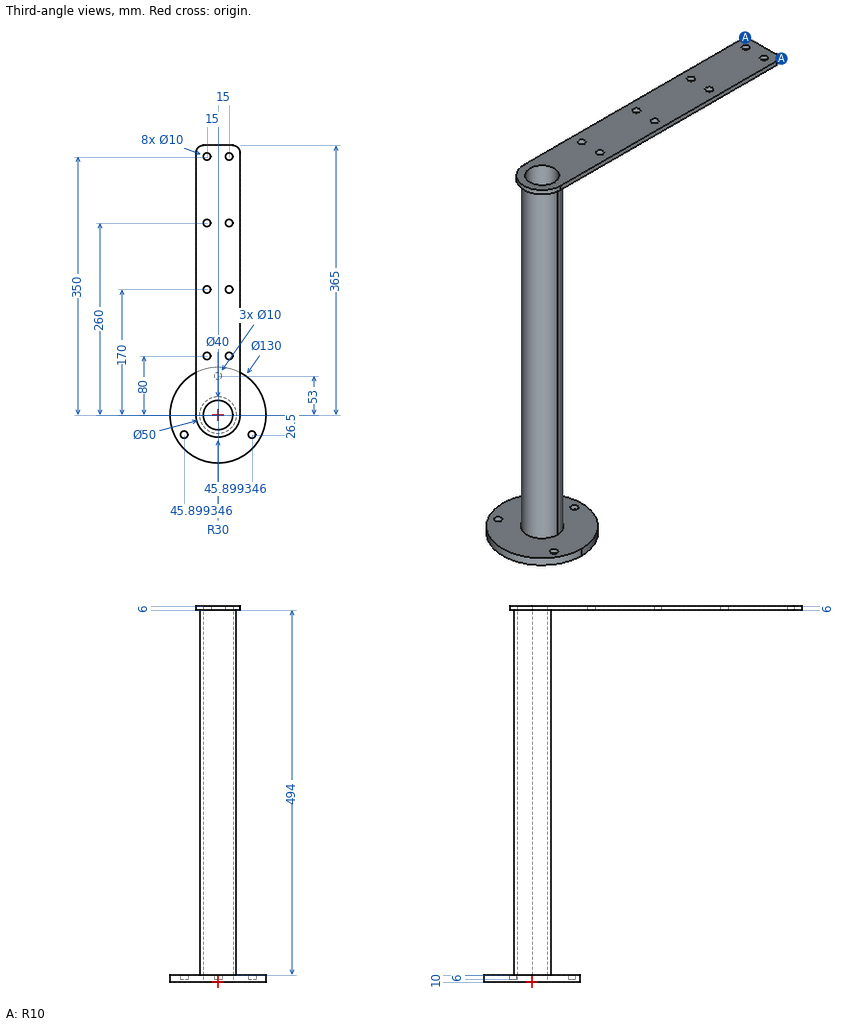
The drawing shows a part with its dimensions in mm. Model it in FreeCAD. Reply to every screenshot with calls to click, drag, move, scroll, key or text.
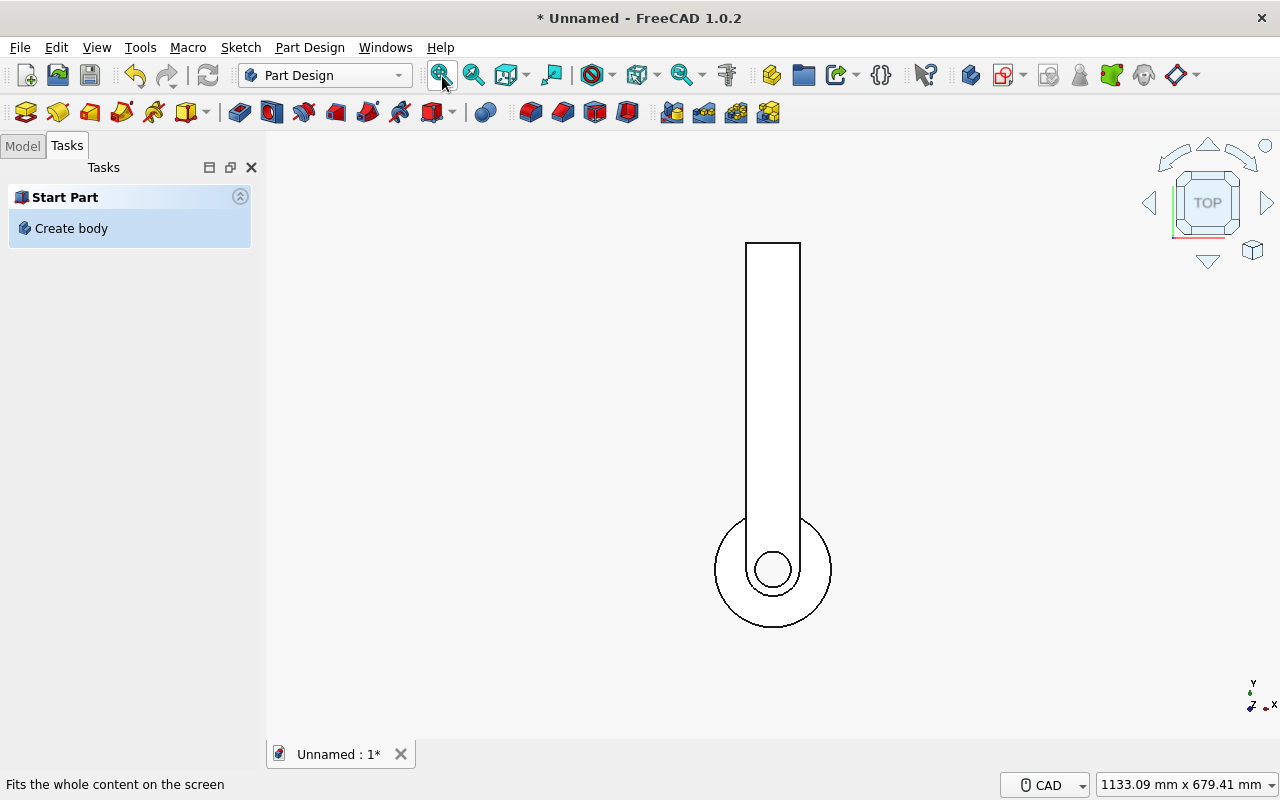
scroll(800, 242, up, 11)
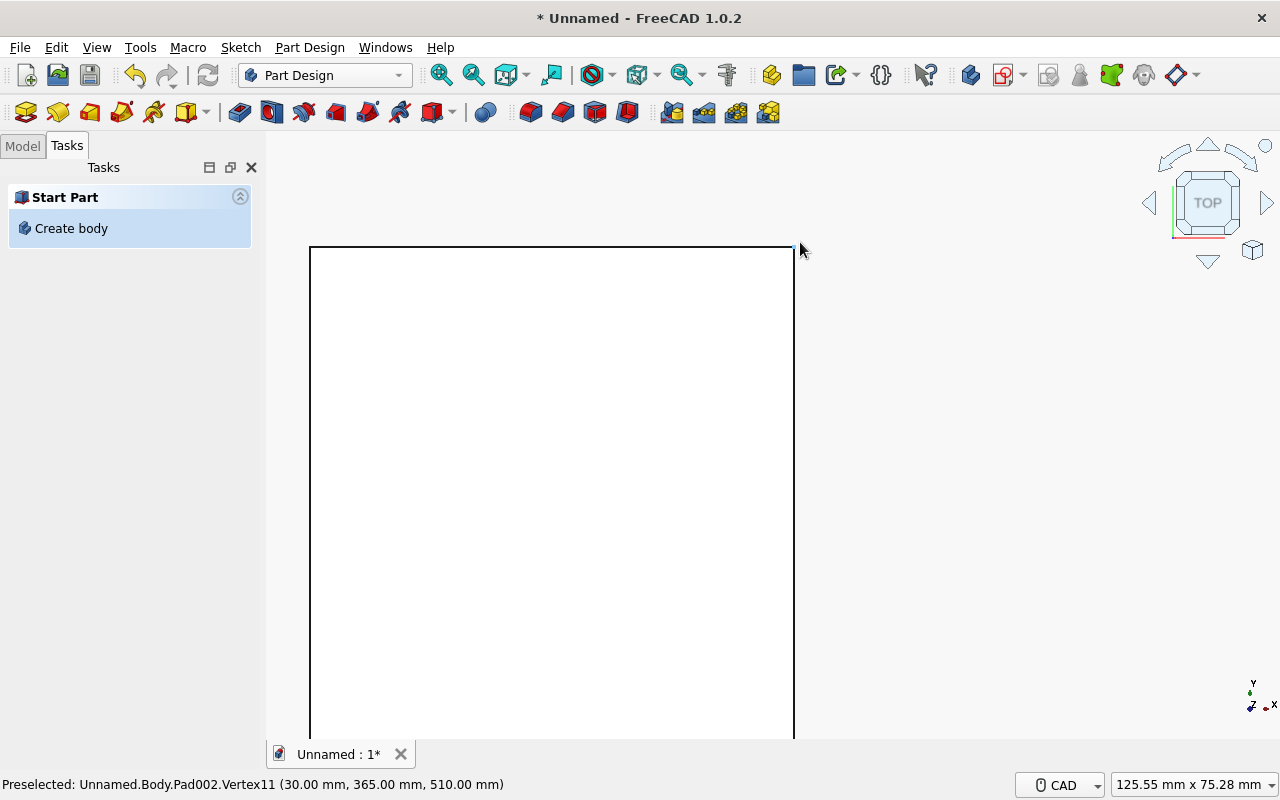
click(442, 76)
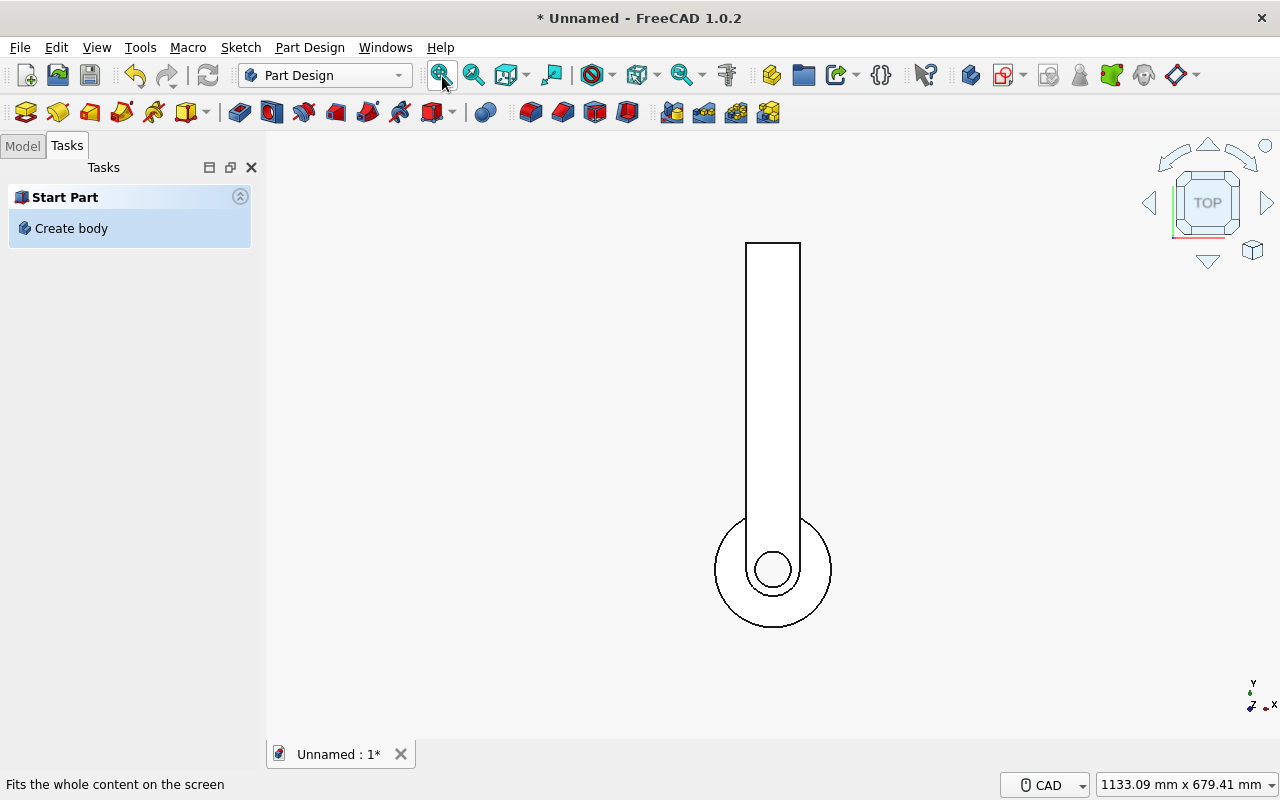
key(1)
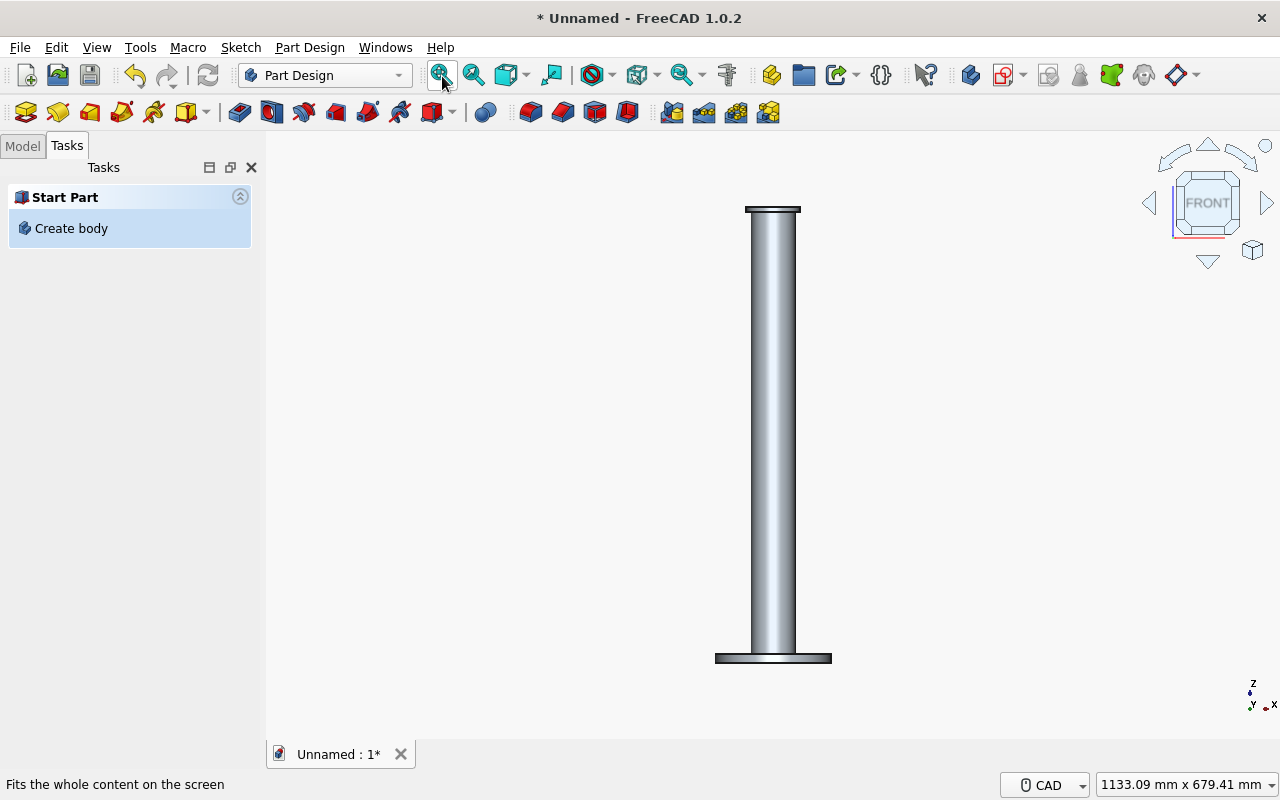
scroll(800, 208, up, 11)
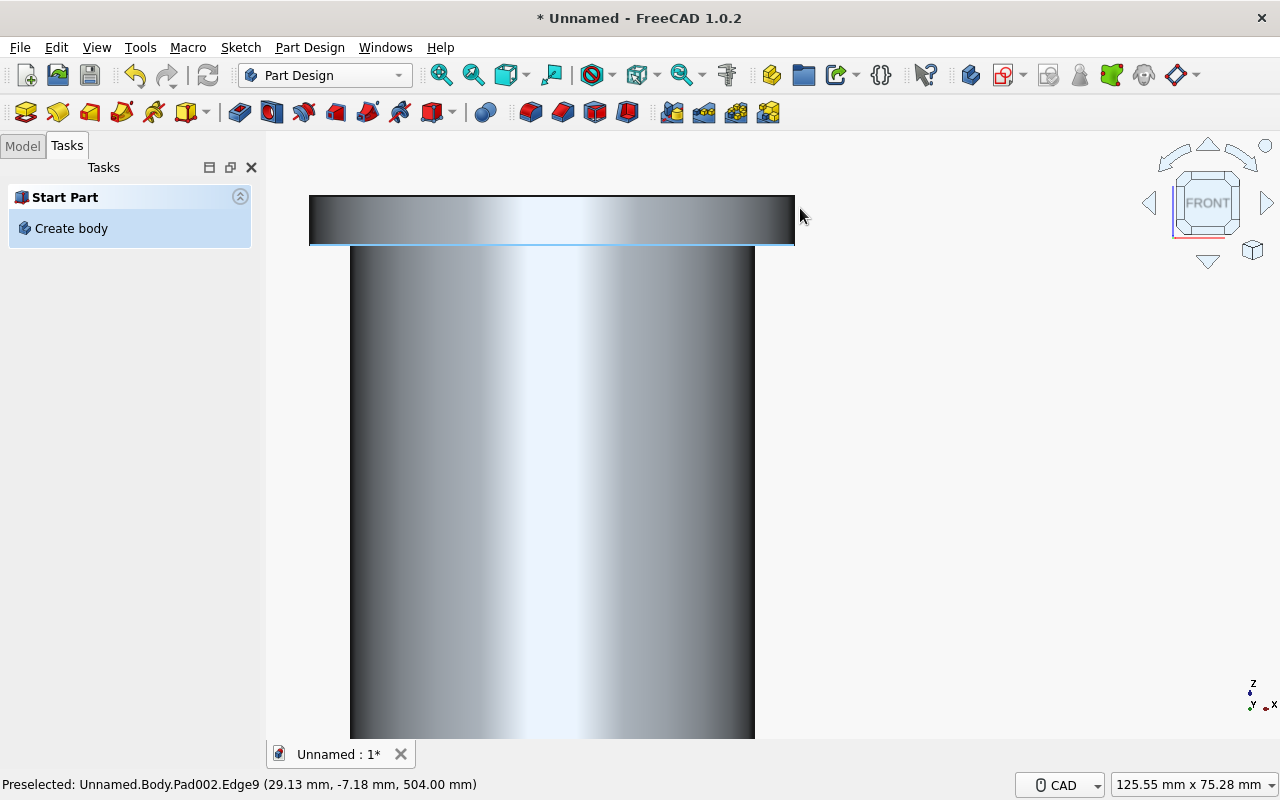
click(442, 76)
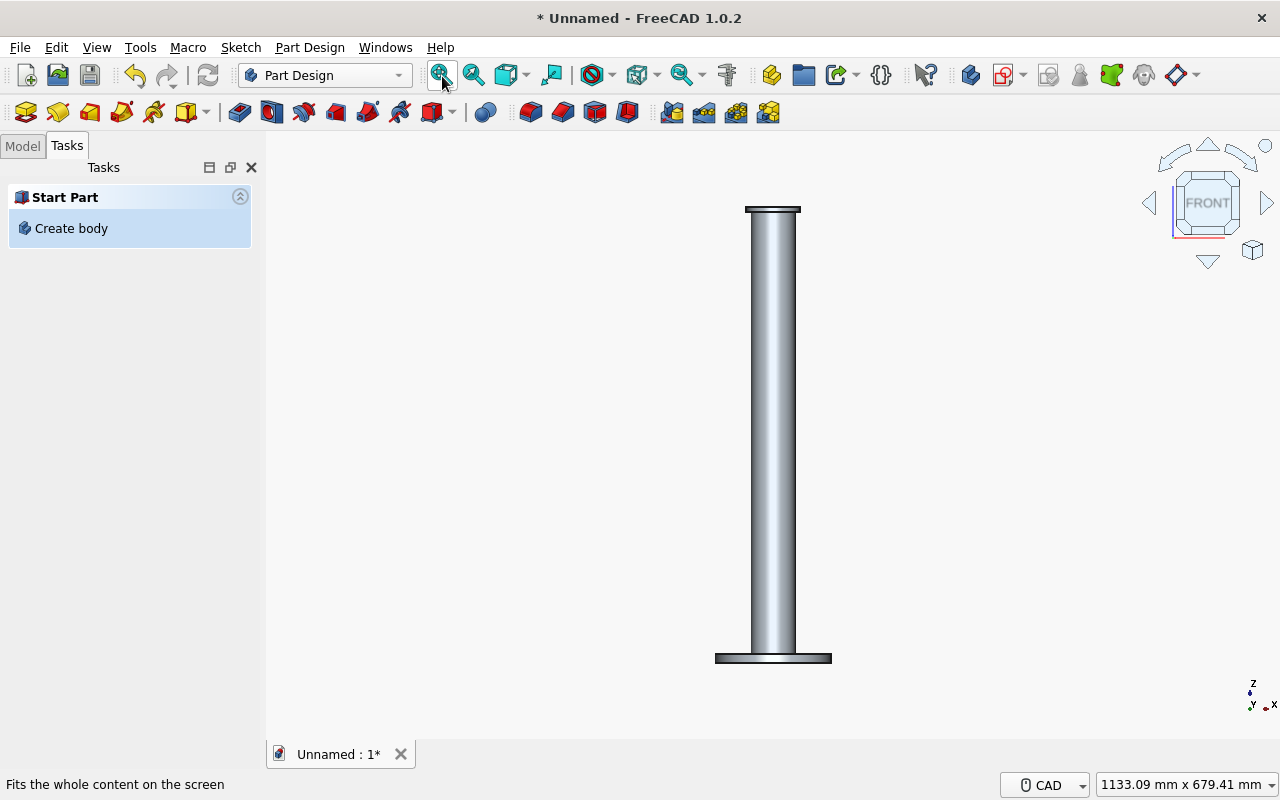
key(3)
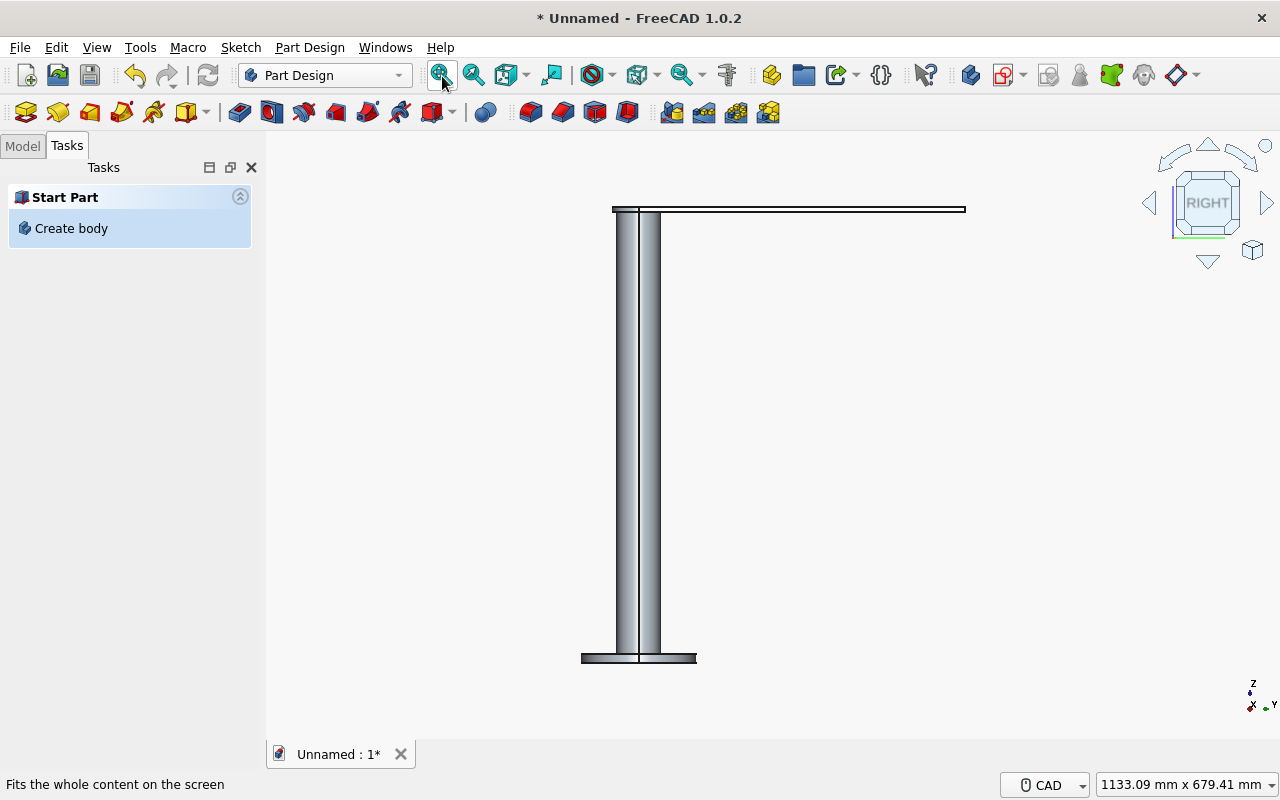
scroll(965, 208, up, 11)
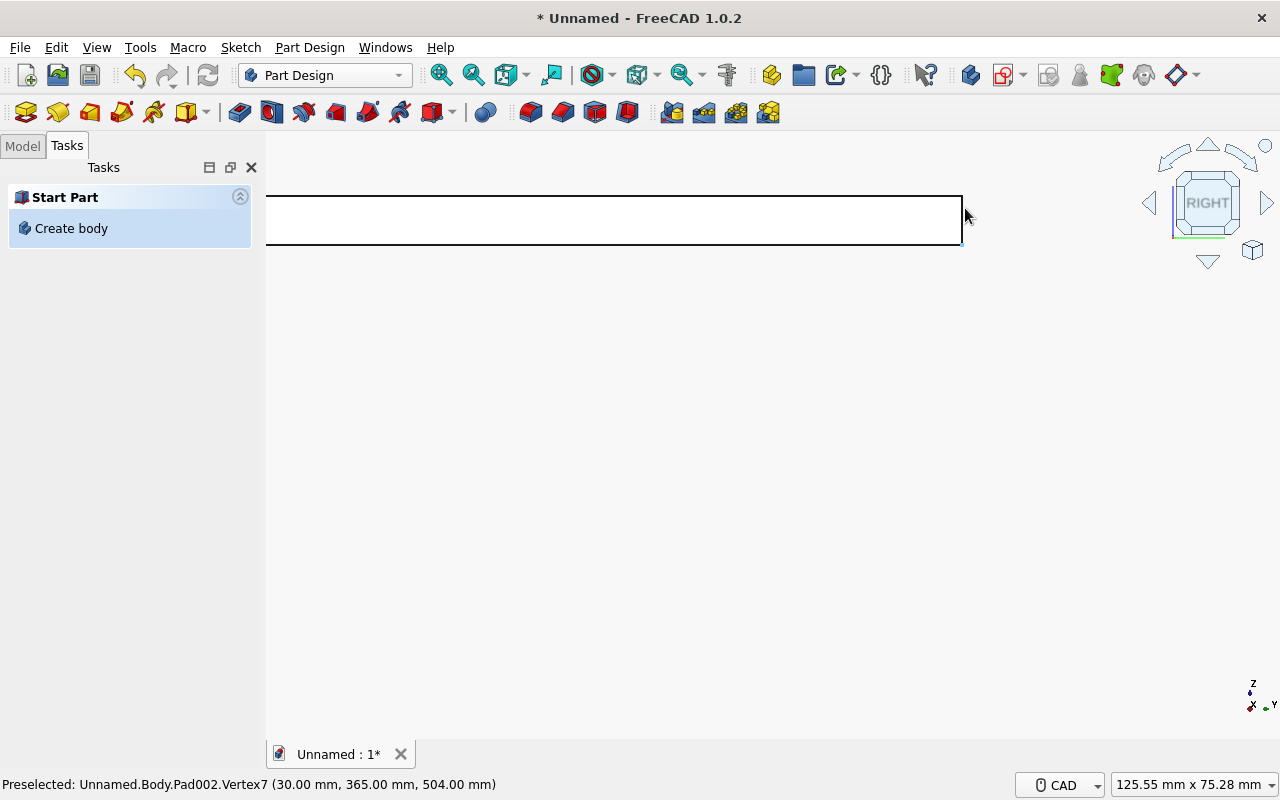
click(962, 219)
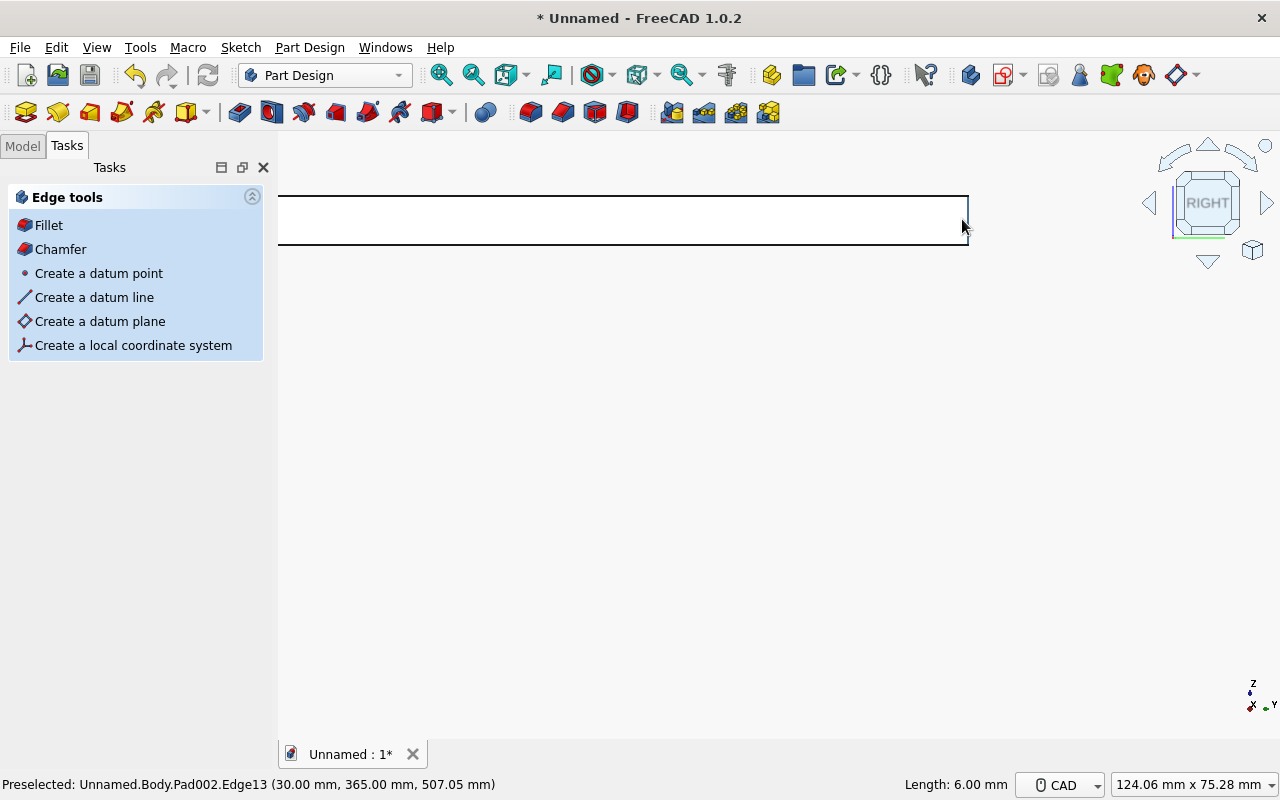
click(442, 76)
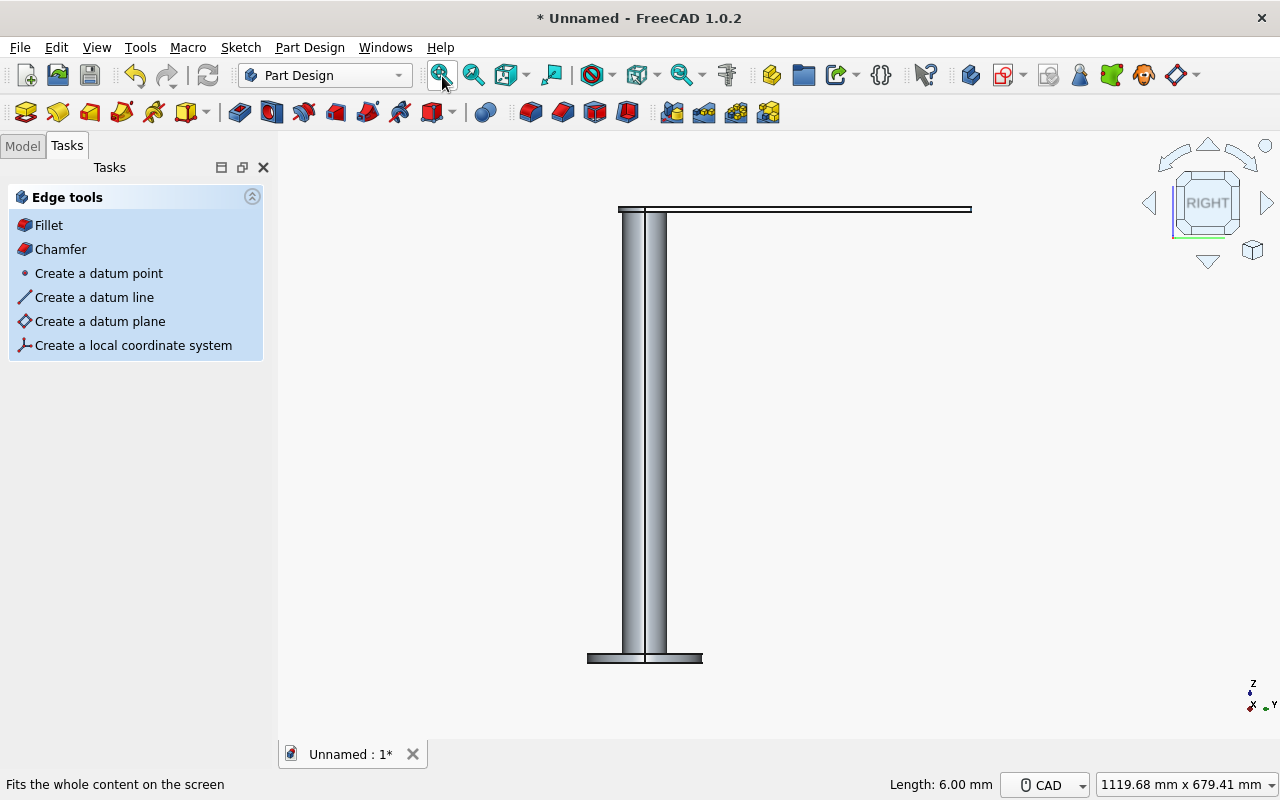
key(5)